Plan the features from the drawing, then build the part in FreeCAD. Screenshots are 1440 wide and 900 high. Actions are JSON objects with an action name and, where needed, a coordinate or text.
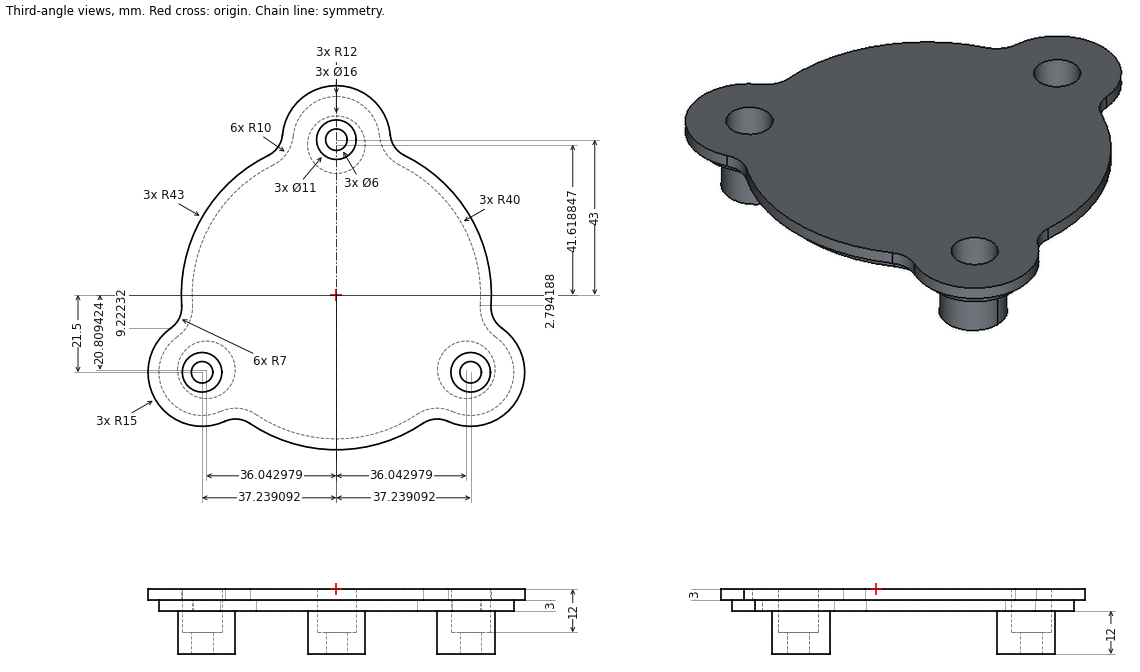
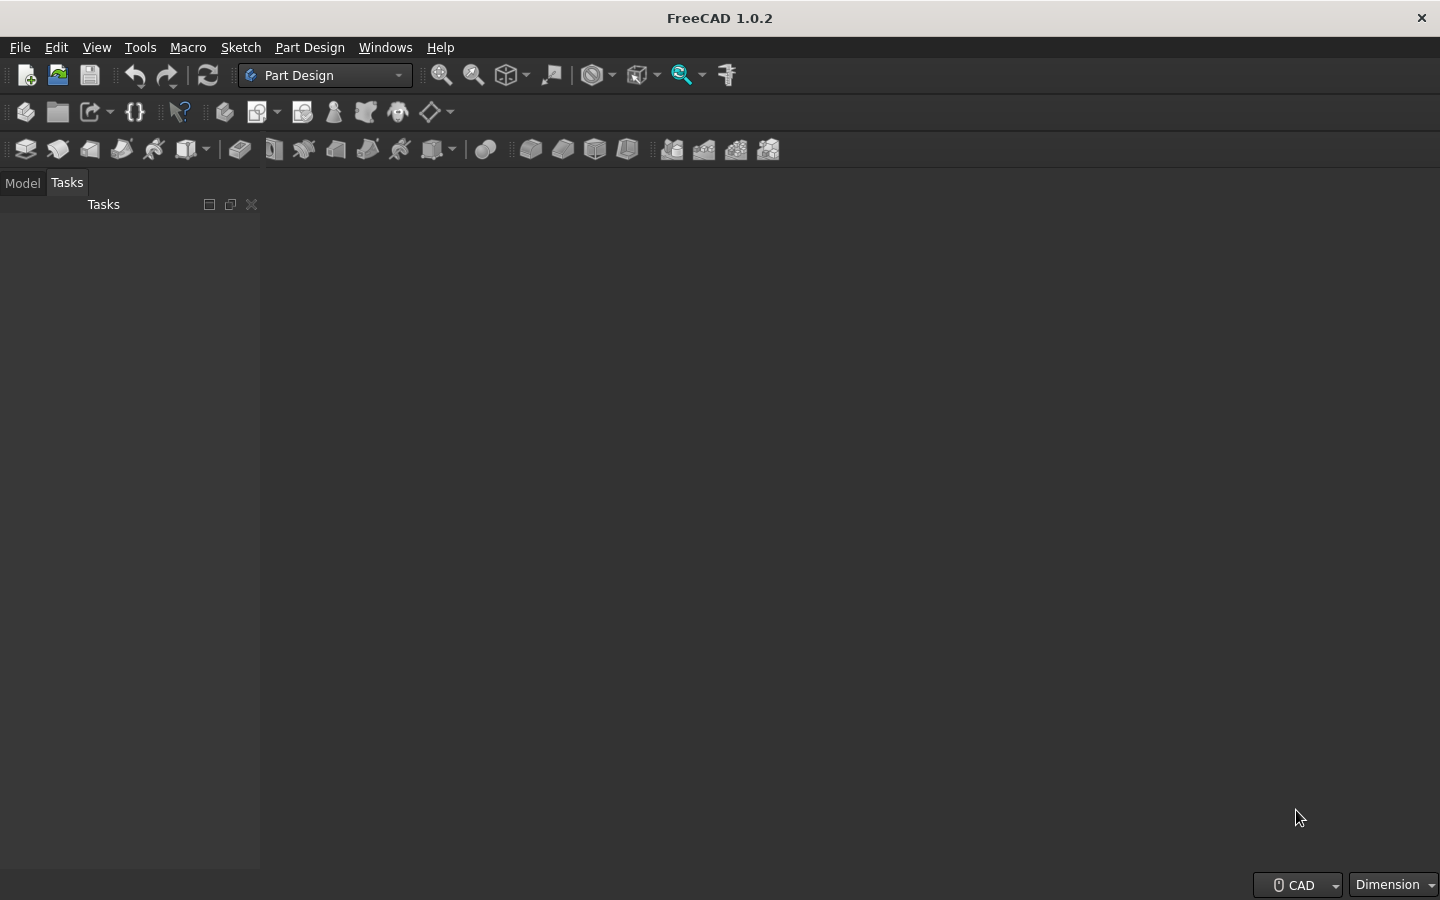
{"action": "left_click", "coordinate": [26, 76]}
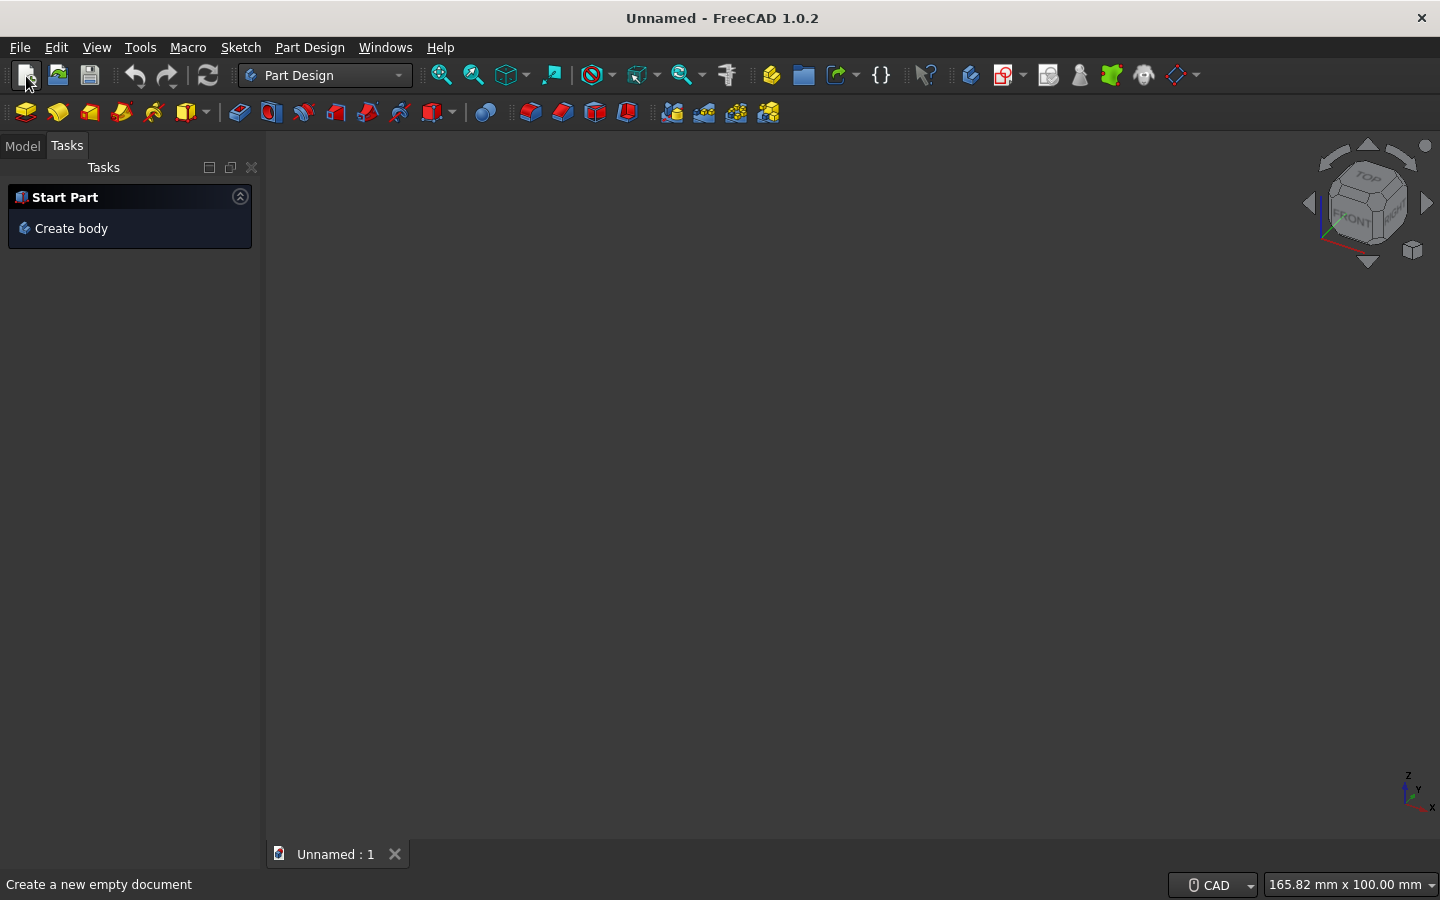
{"action": "left_click", "coordinate": [1004, 76]}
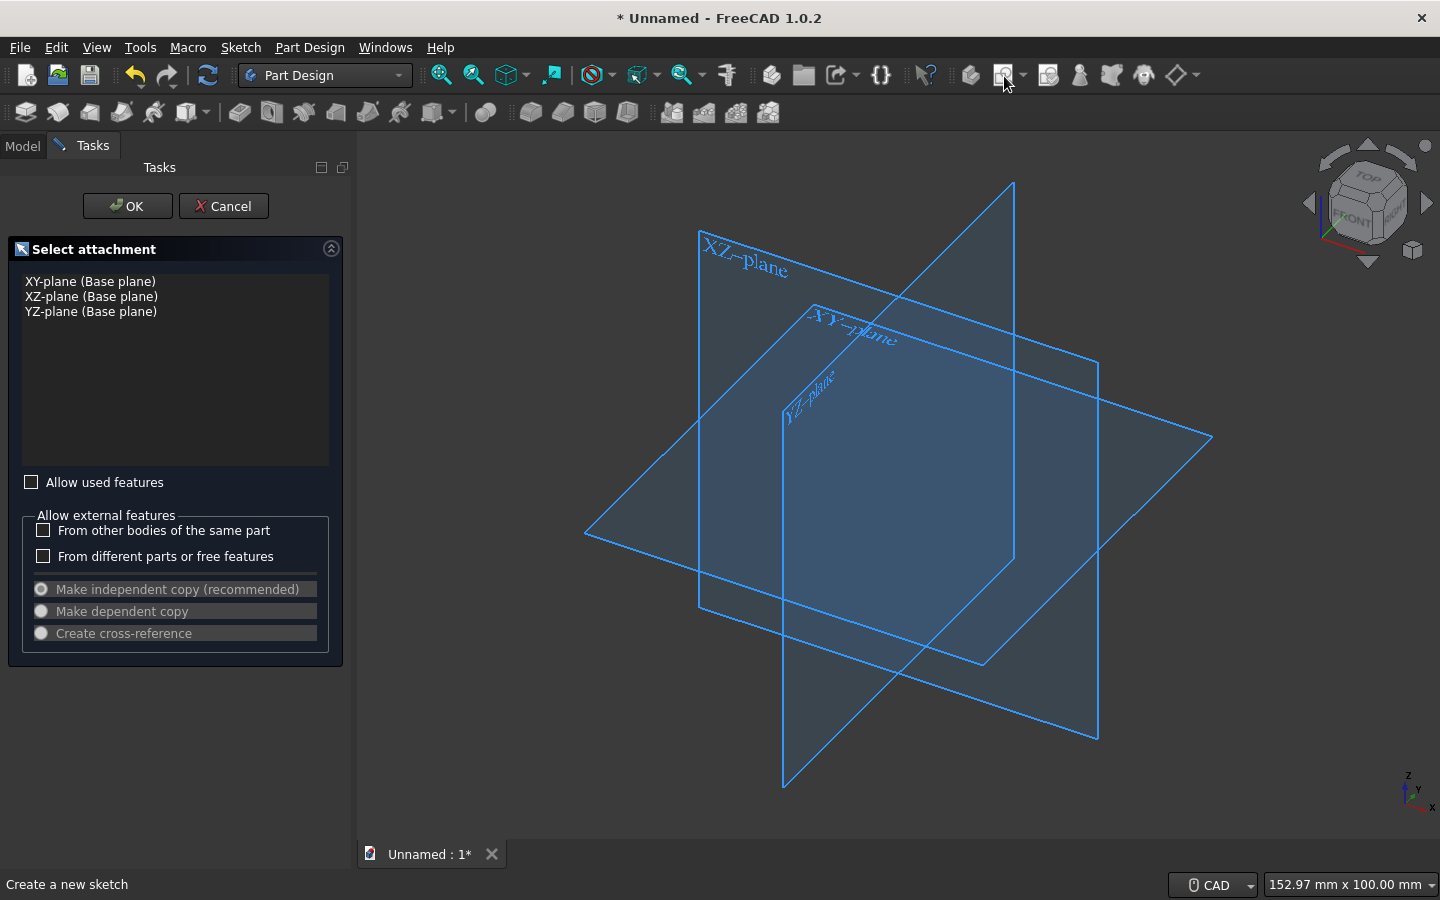
{"action": "left_click", "coordinate": [82, 282]}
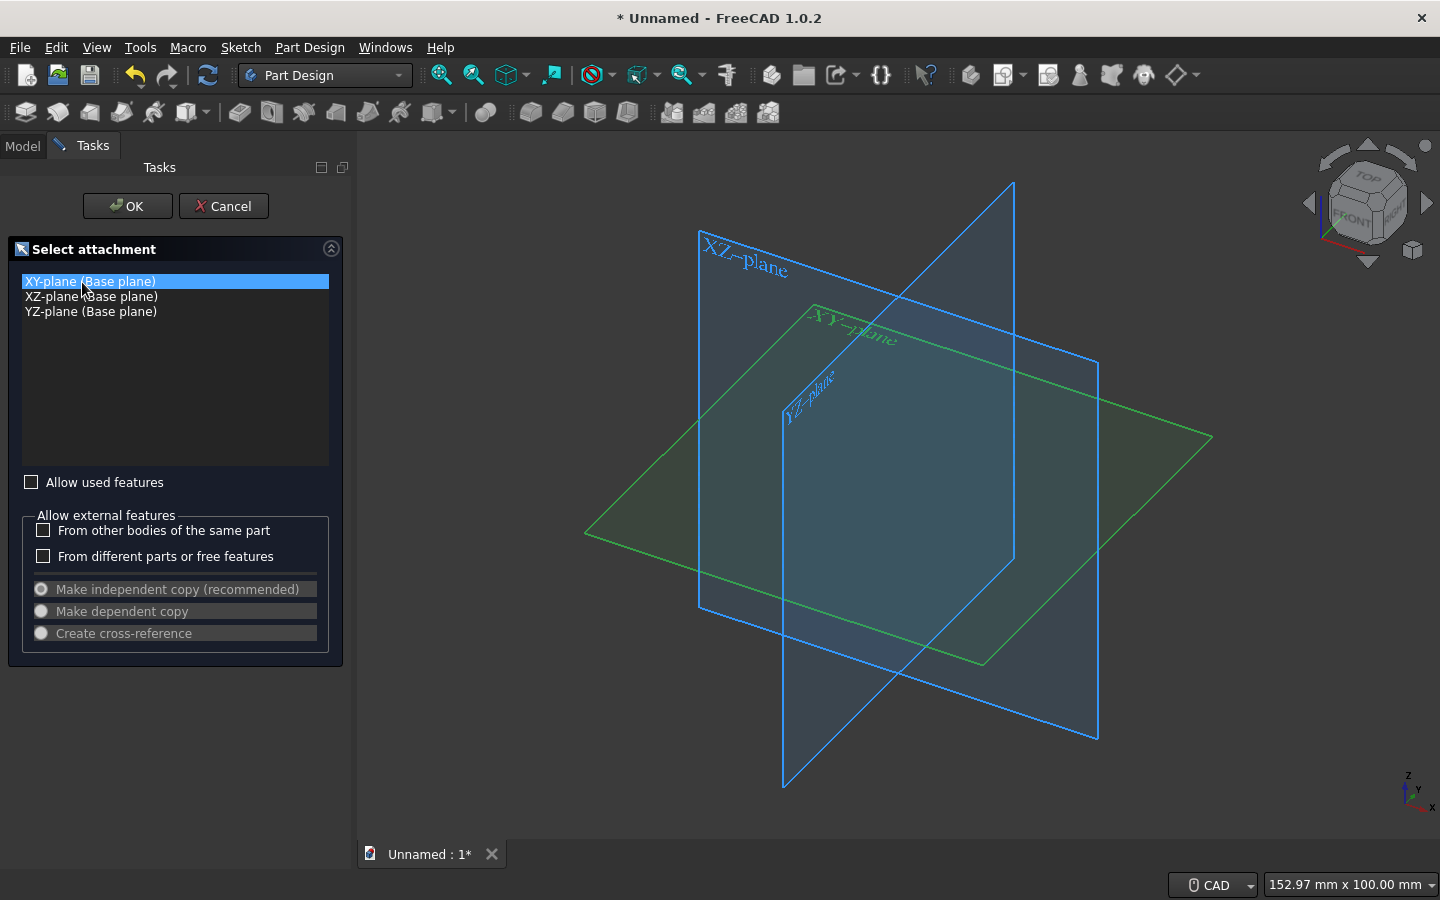
{"action": "left_click", "coordinate": [128, 206]}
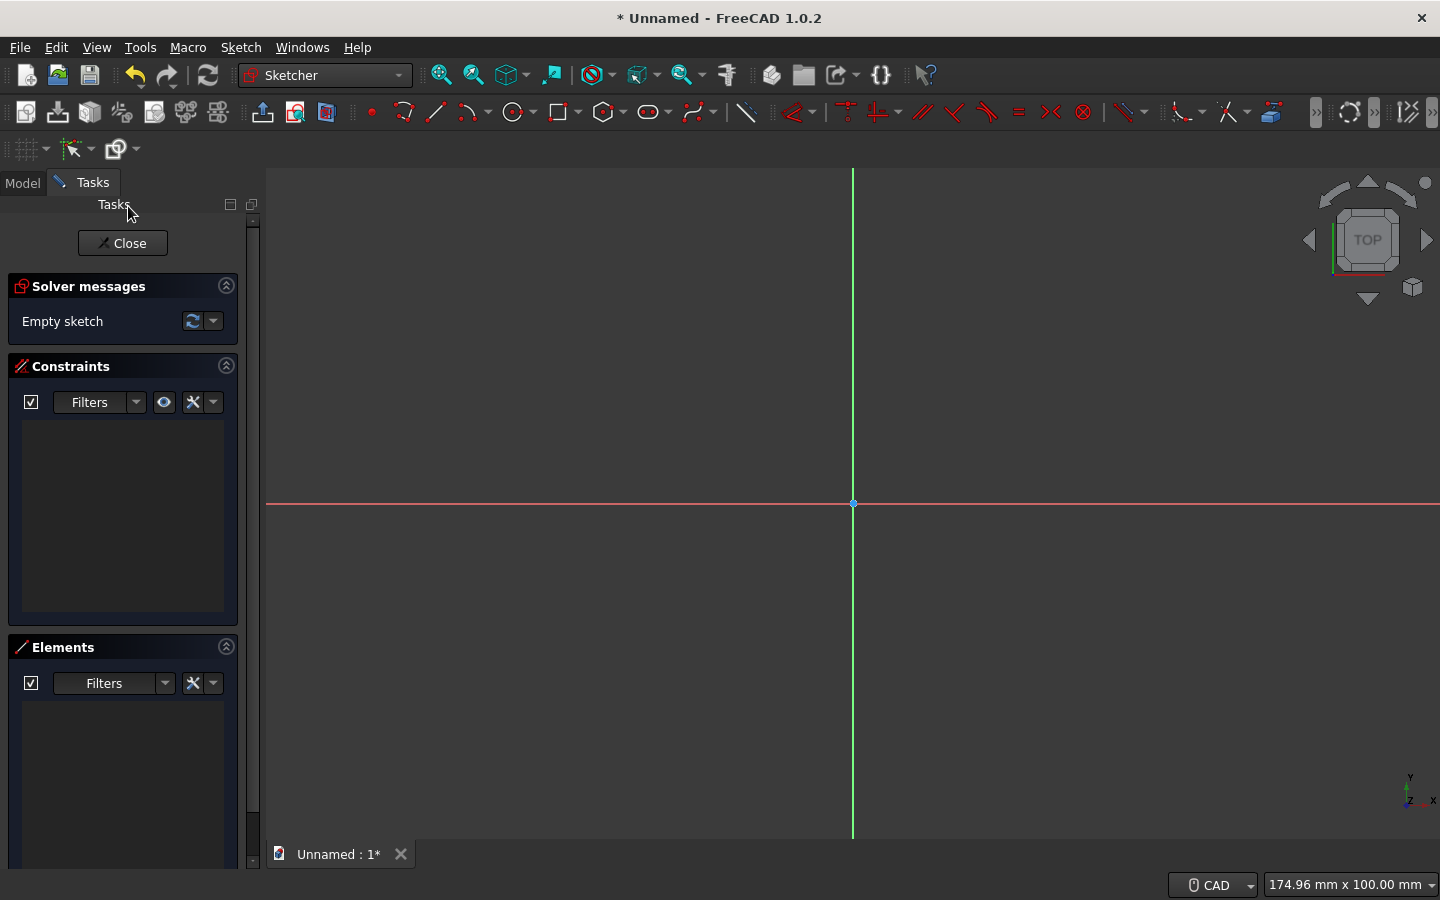
{"action": "scroll", "coordinate": [645, 606], "scroll_direction": "down", "scroll_amount": 2}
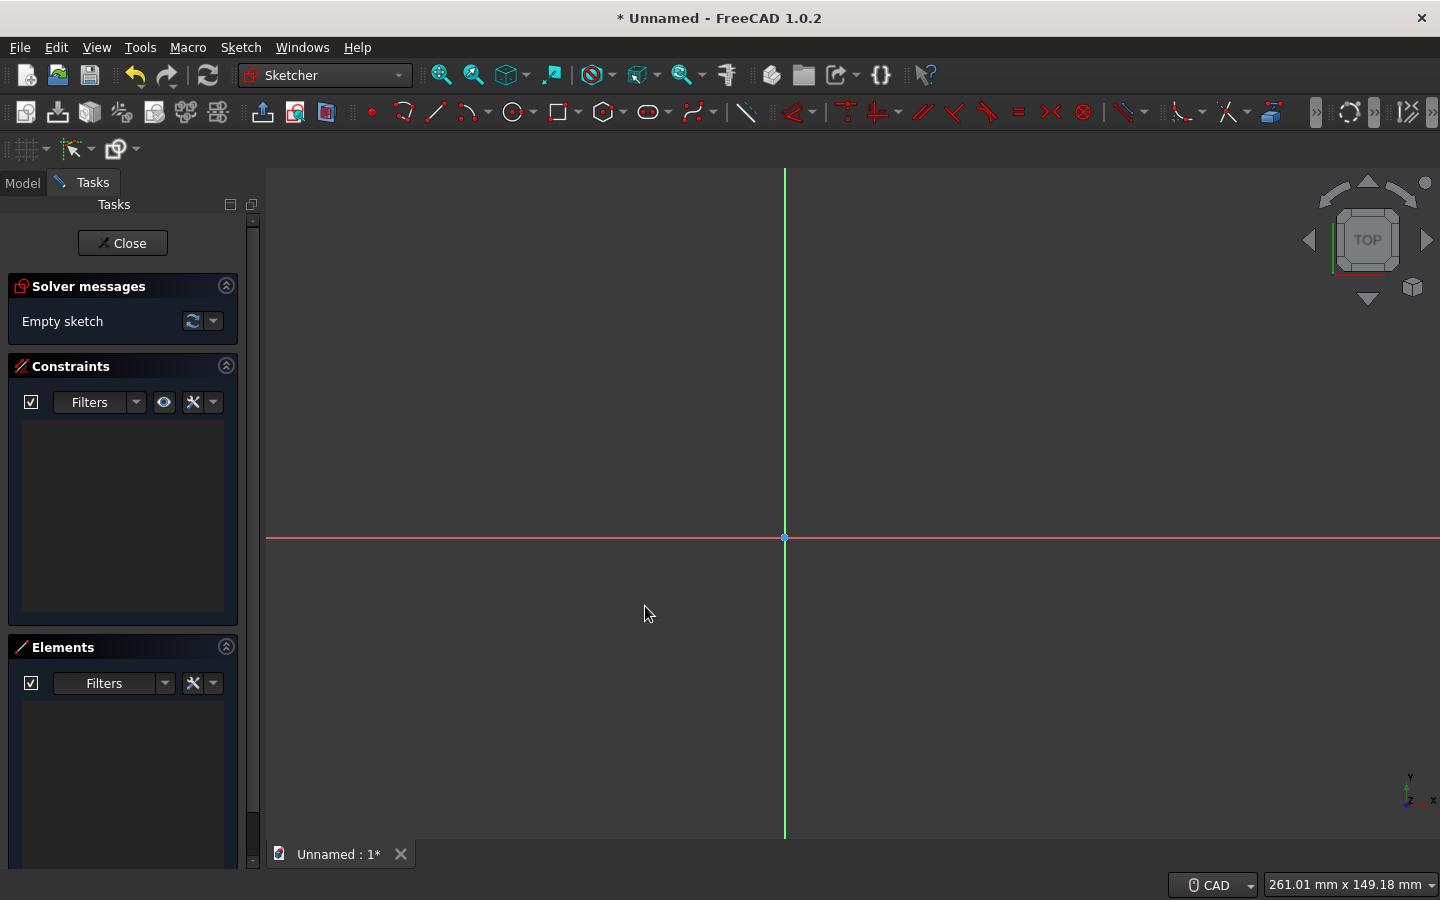
{"action": "left_click", "coordinate": [490, 112]}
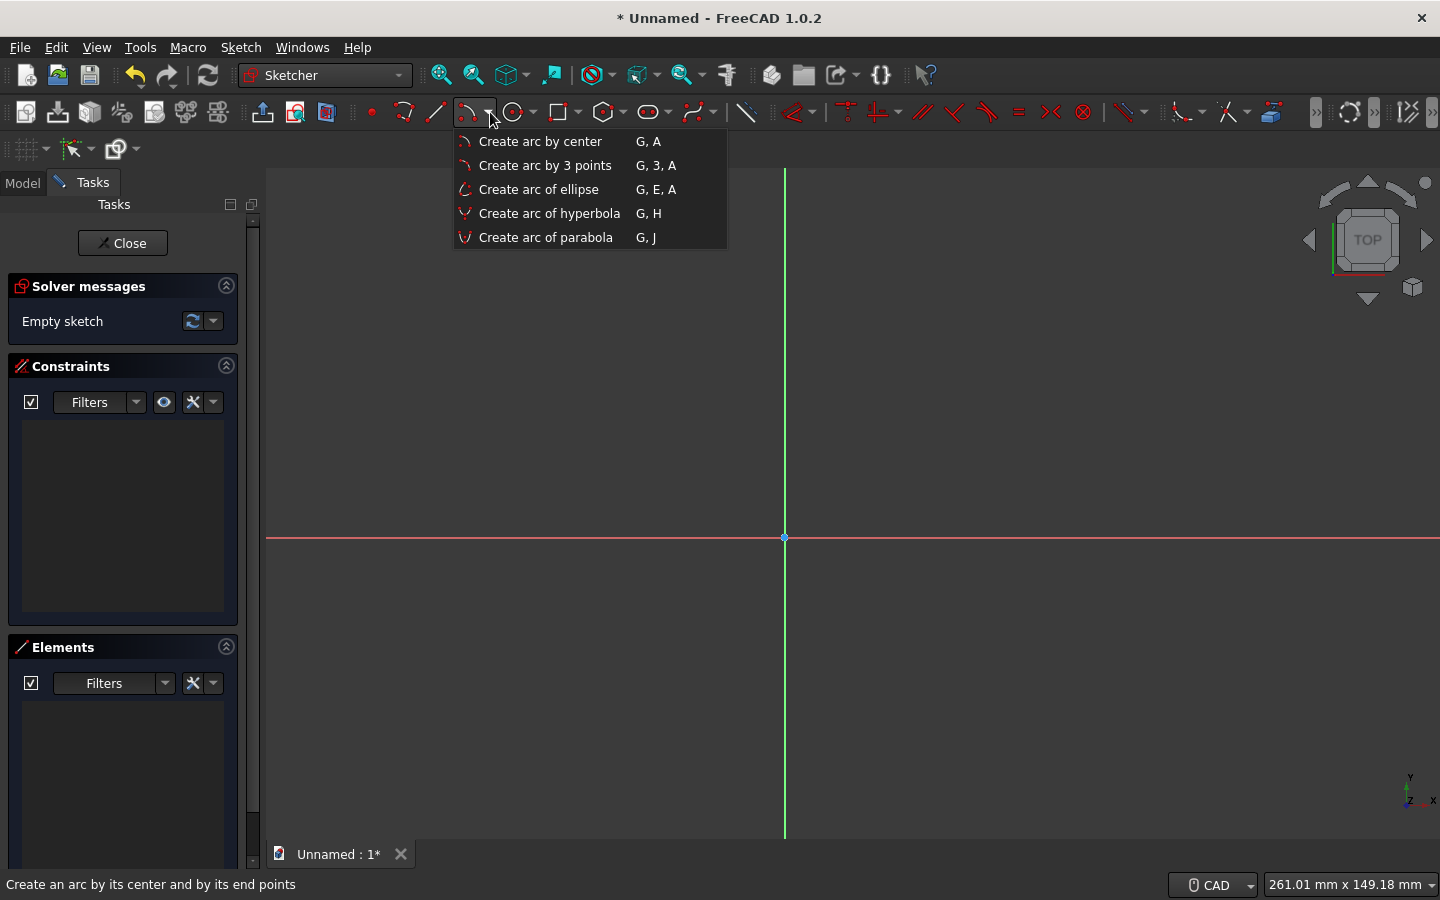
{"action": "left_click", "coordinate": [590, 165]}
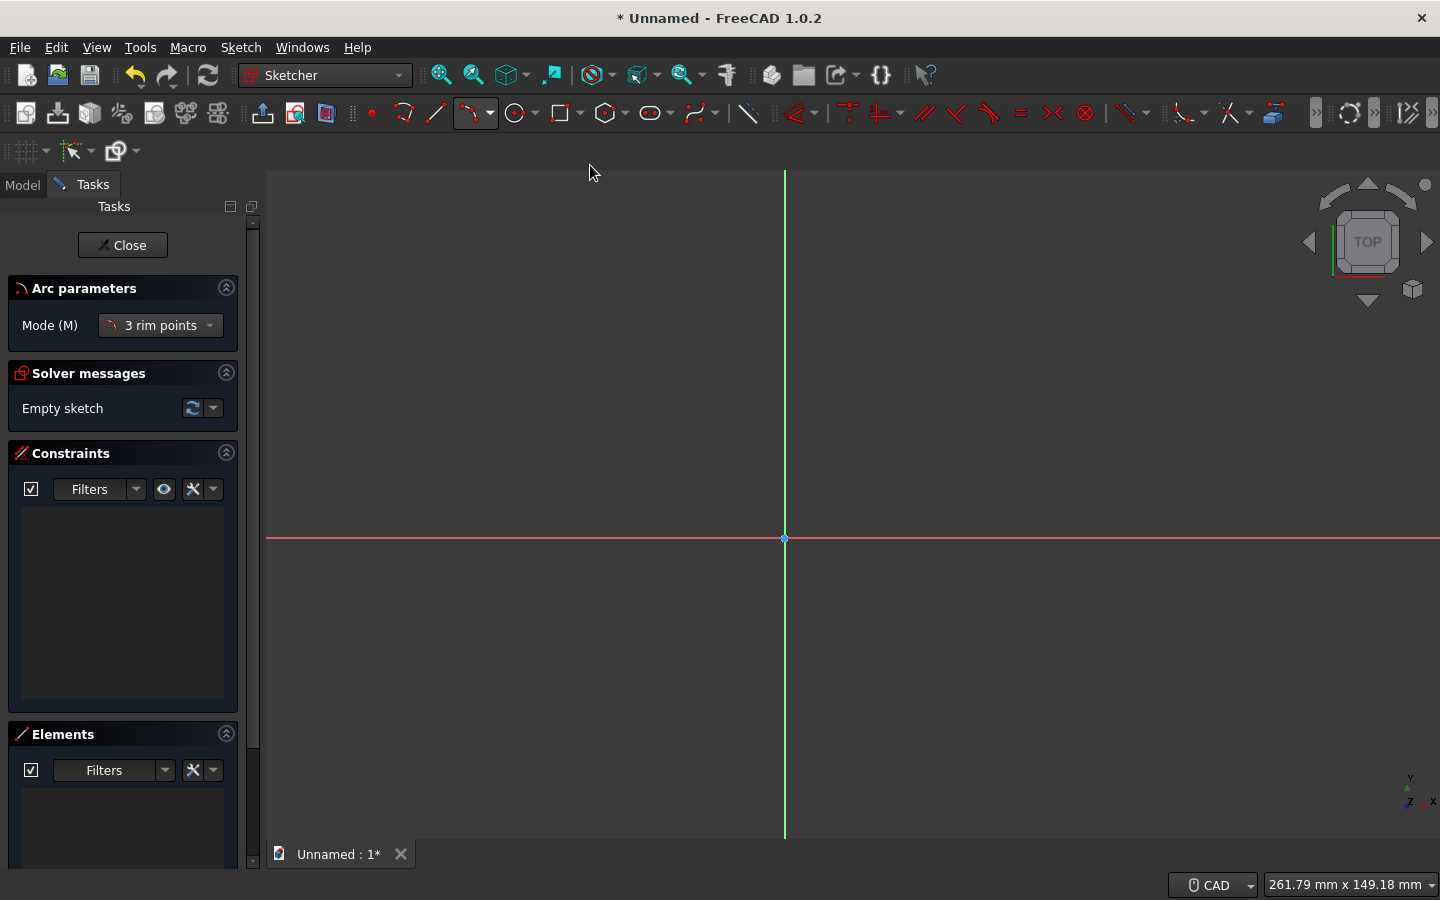
{"action": "left_click", "coordinate": [592, 552]}
{"action": "left_click", "coordinate": [579, 580]}